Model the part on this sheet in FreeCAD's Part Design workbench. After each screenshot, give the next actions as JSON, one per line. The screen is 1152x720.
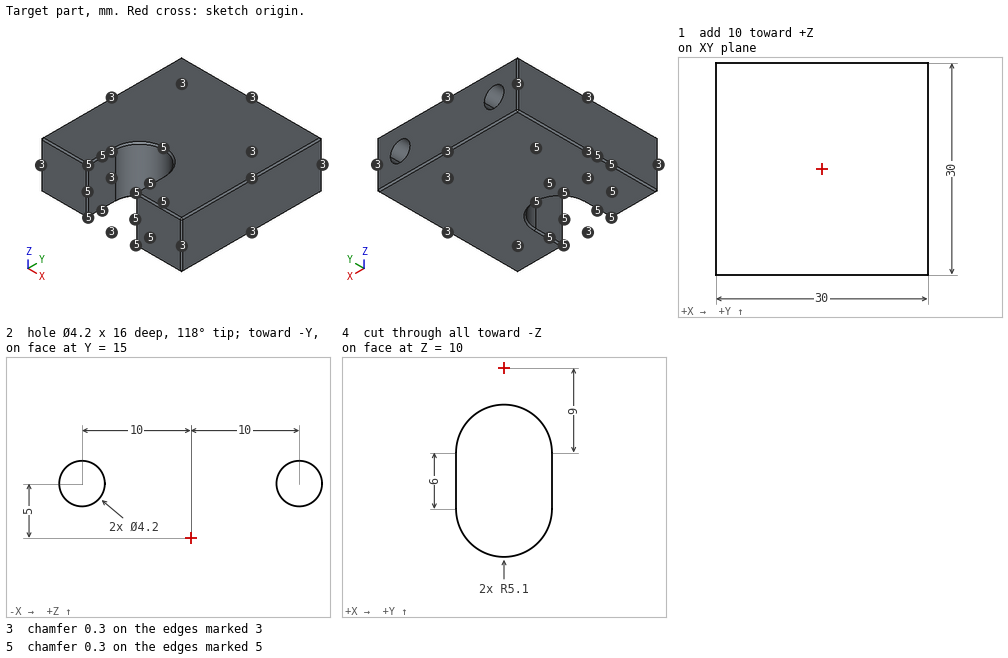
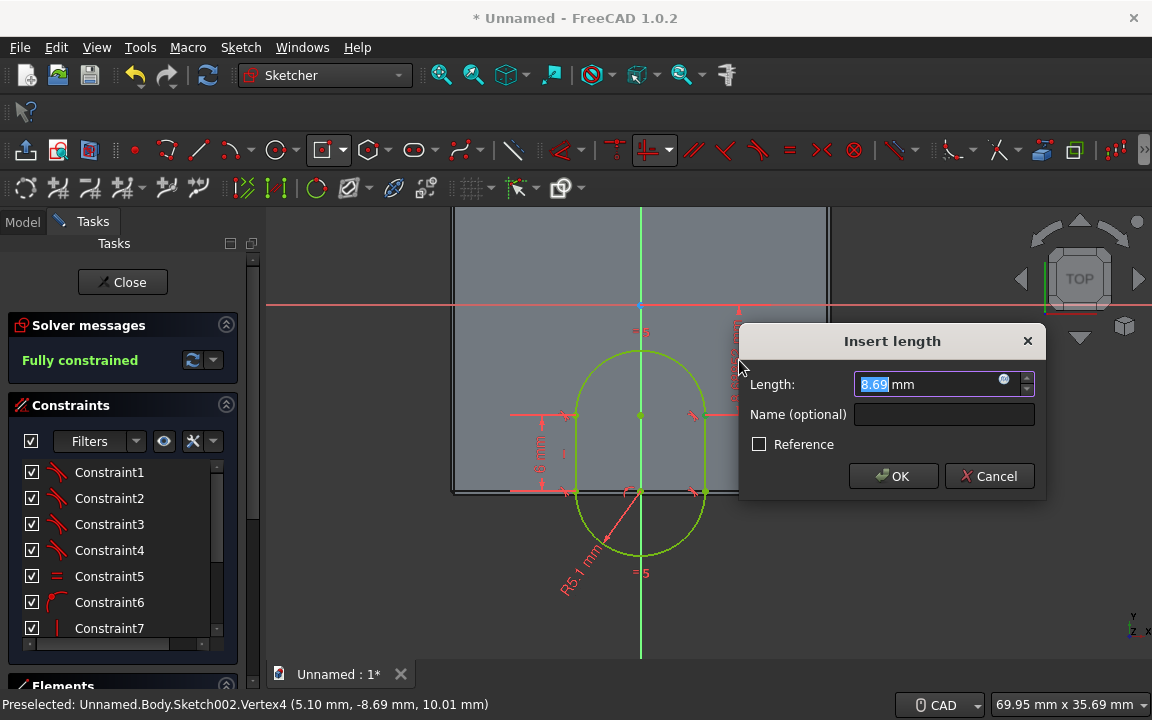
{"action": "type", "text": "9"}
{"action": "key", "text": "Return"}
{"action": "key", "text": "Escape"}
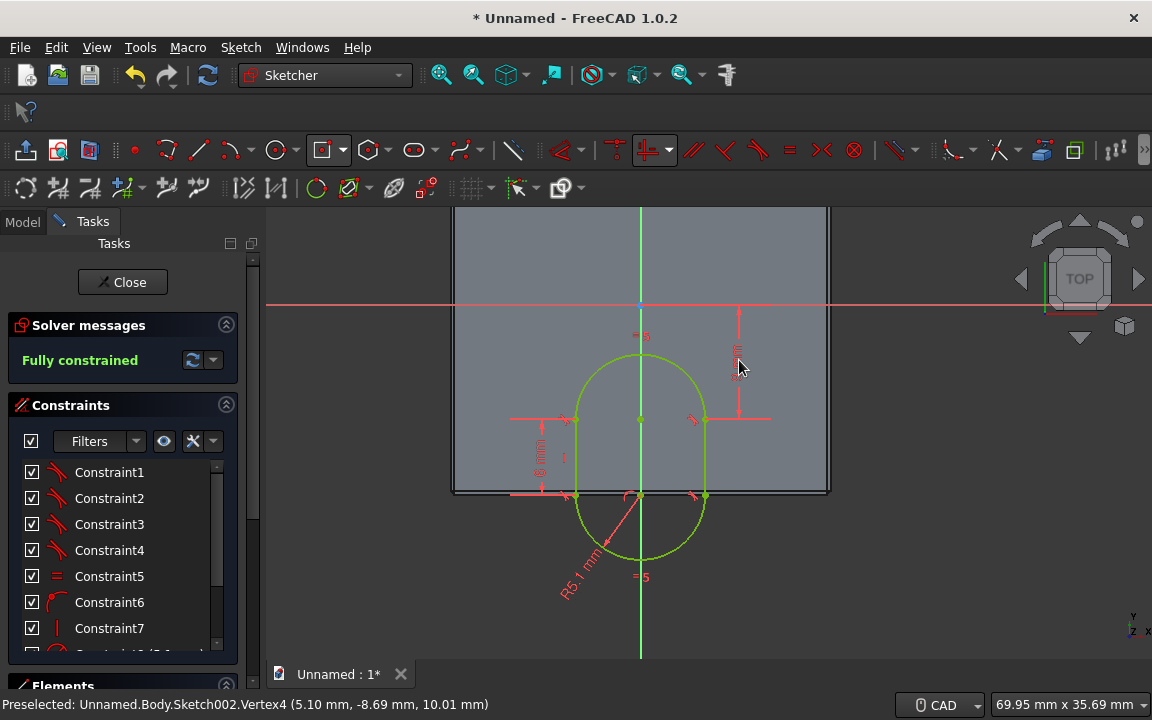
{"action": "left_click", "coordinate": [123, 282]}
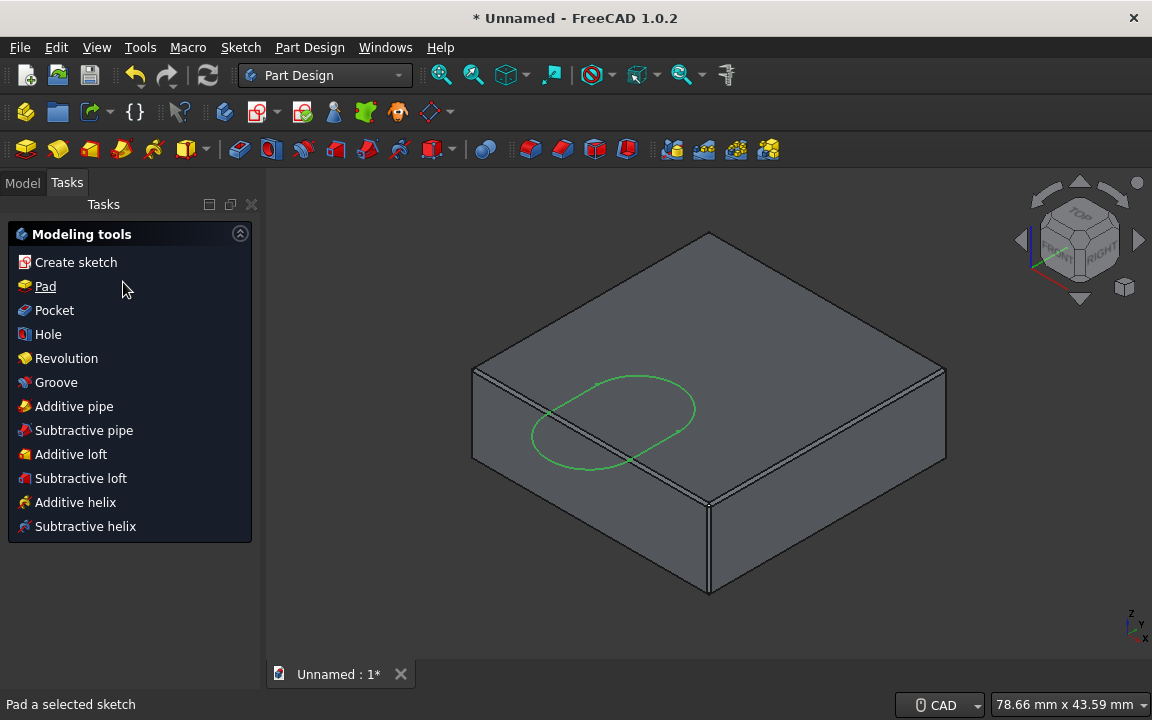
{"action": "left_click", "coordinate": [240, 150]}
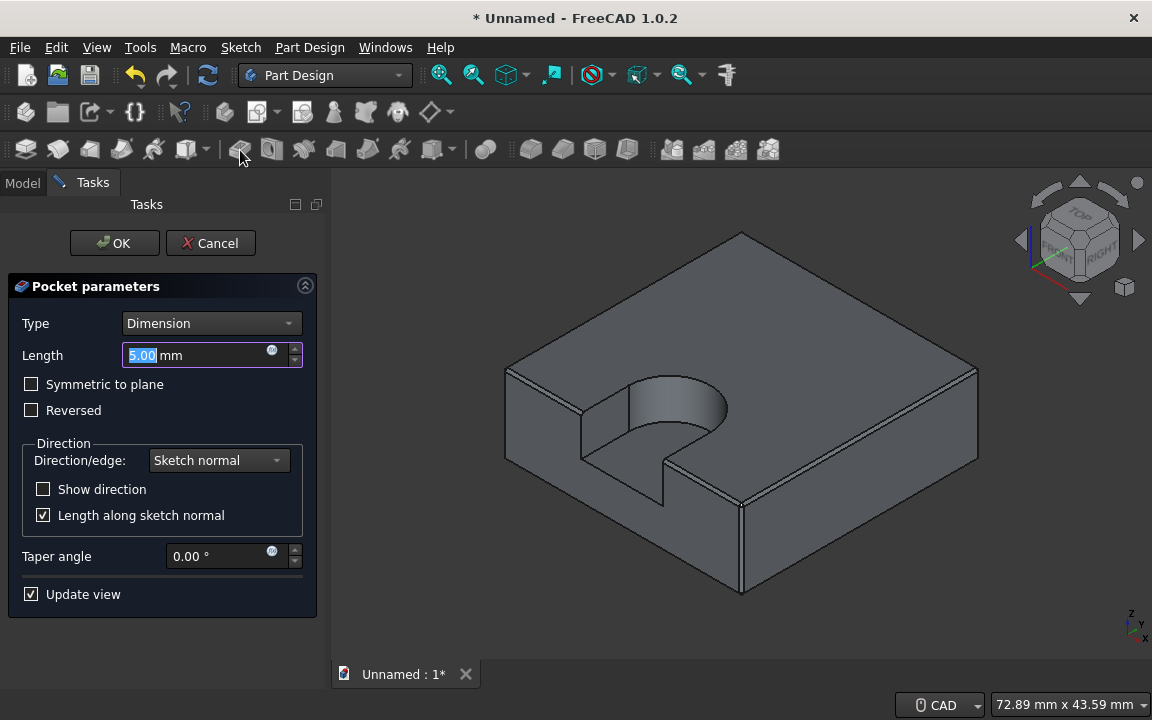
{"action": "left_click", "coordinate": [212, 324]}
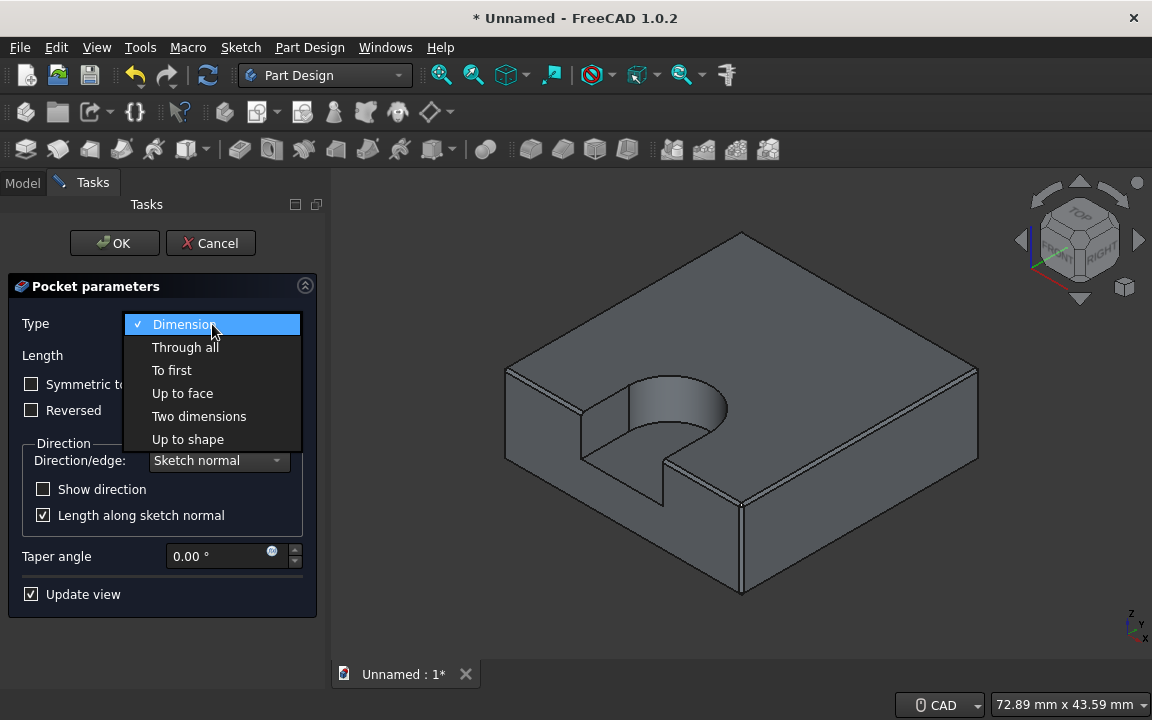
{"action": "left_click", "coordinate": [212, 348]}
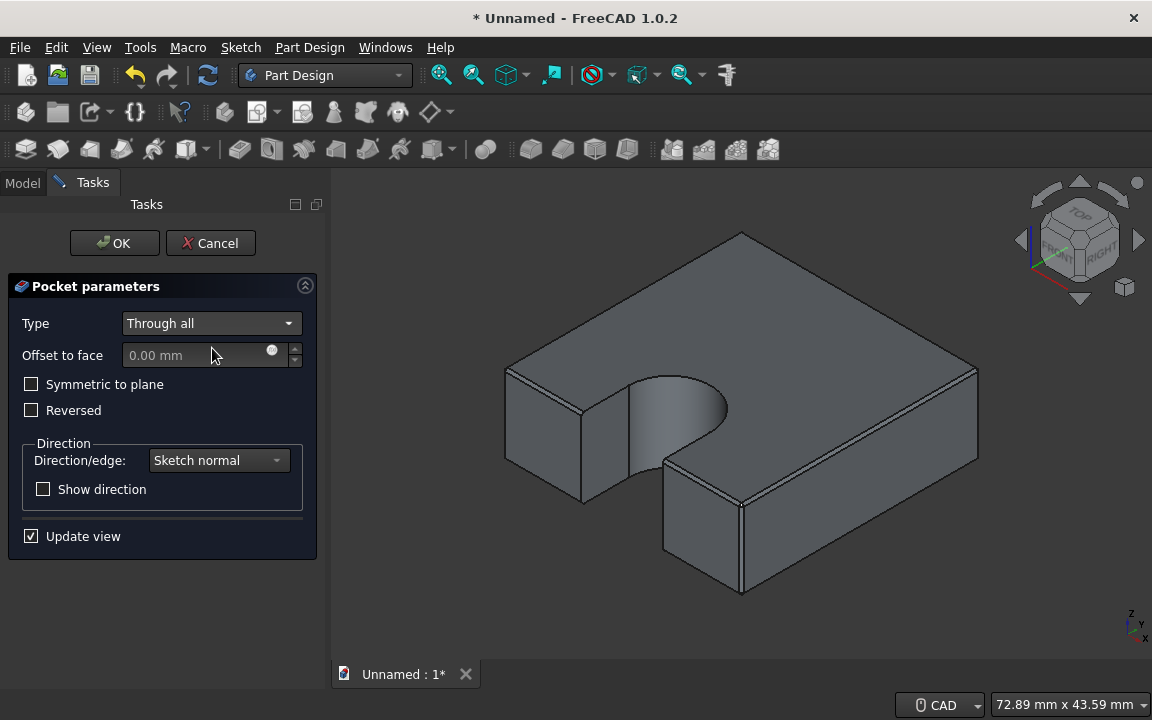
{"action": "left_click", "coordinate": [115, 243]}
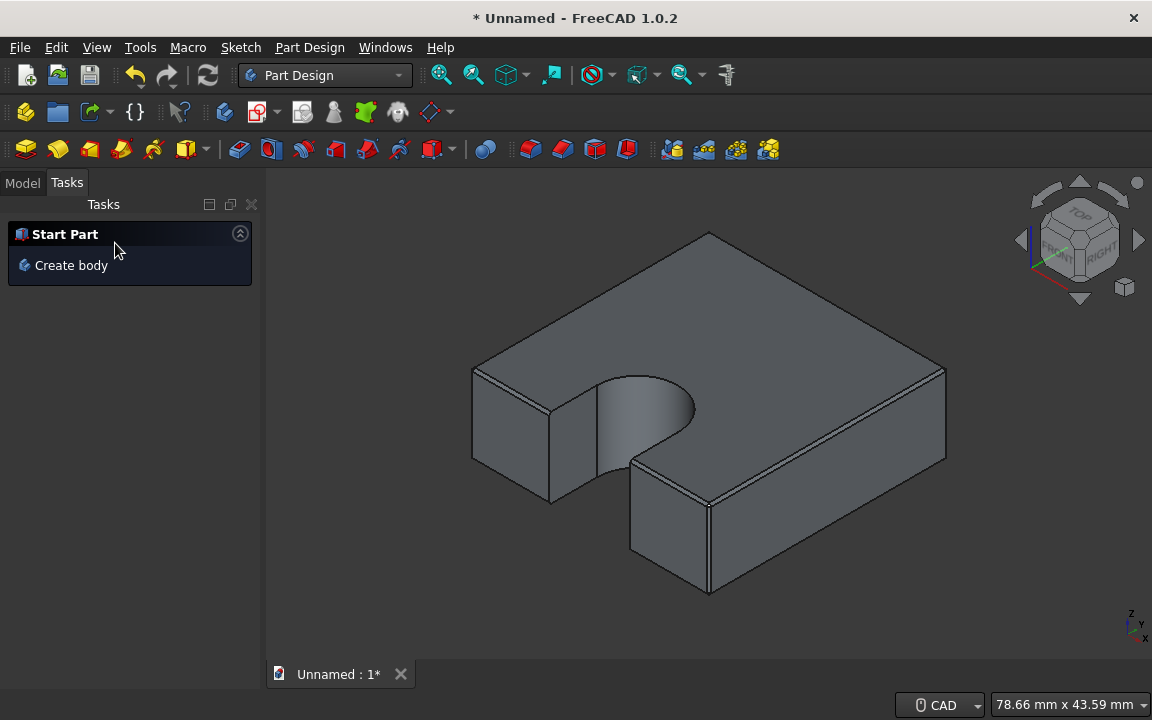
{"action": "left_click", "coordinate": [549, 458]}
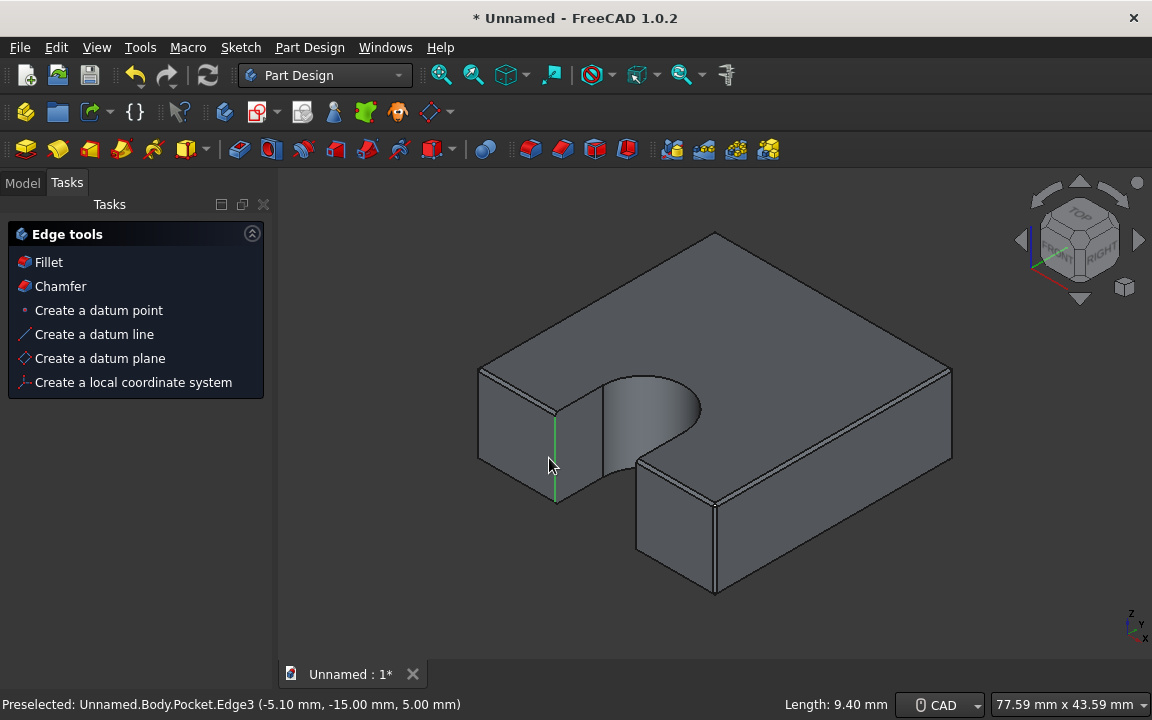
{"action": "left_click", "coordinate": [684, 384], "text": "ctrl"}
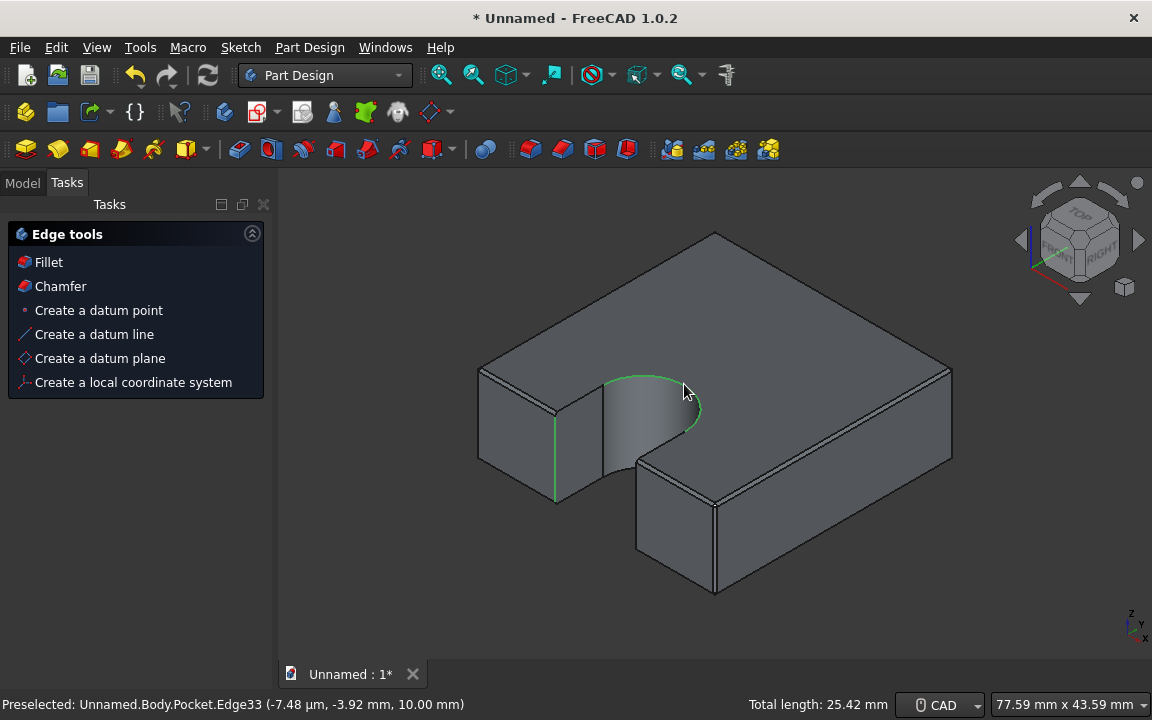
{"action": "left_click", "coordinate": [580, 398], "text": "ctrl"}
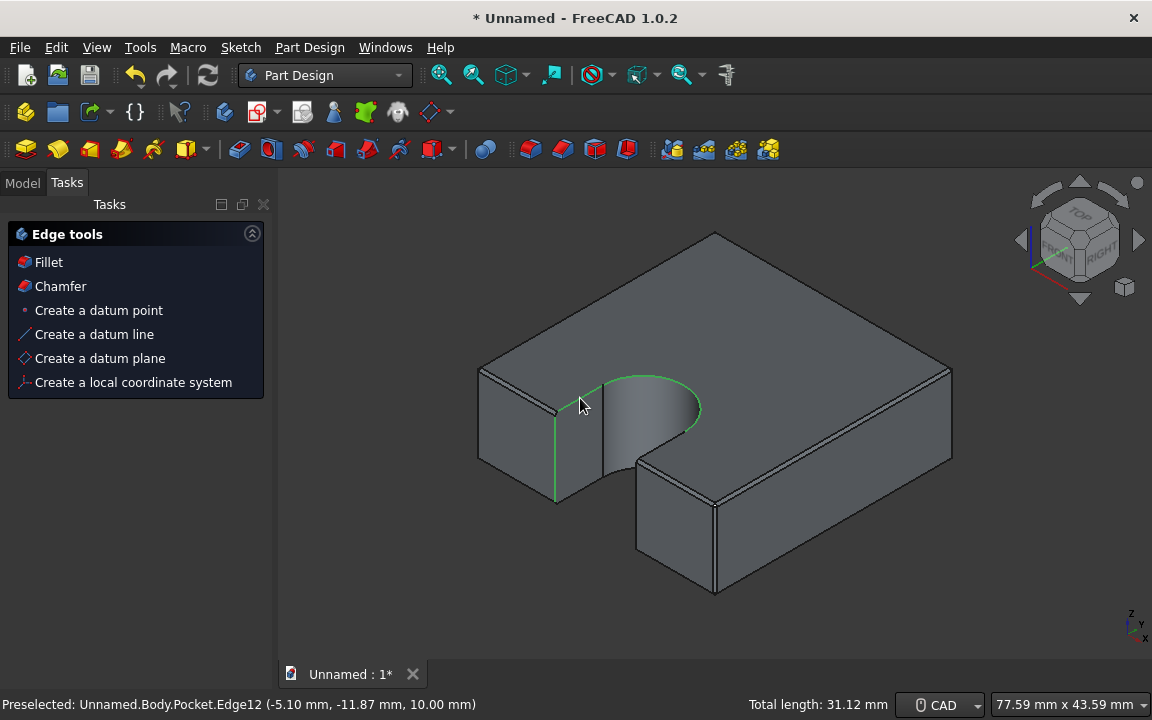
{"action": "scroll", "coordinate": [637, 549], "scroll_direction": "up", "scroll_amount": 11}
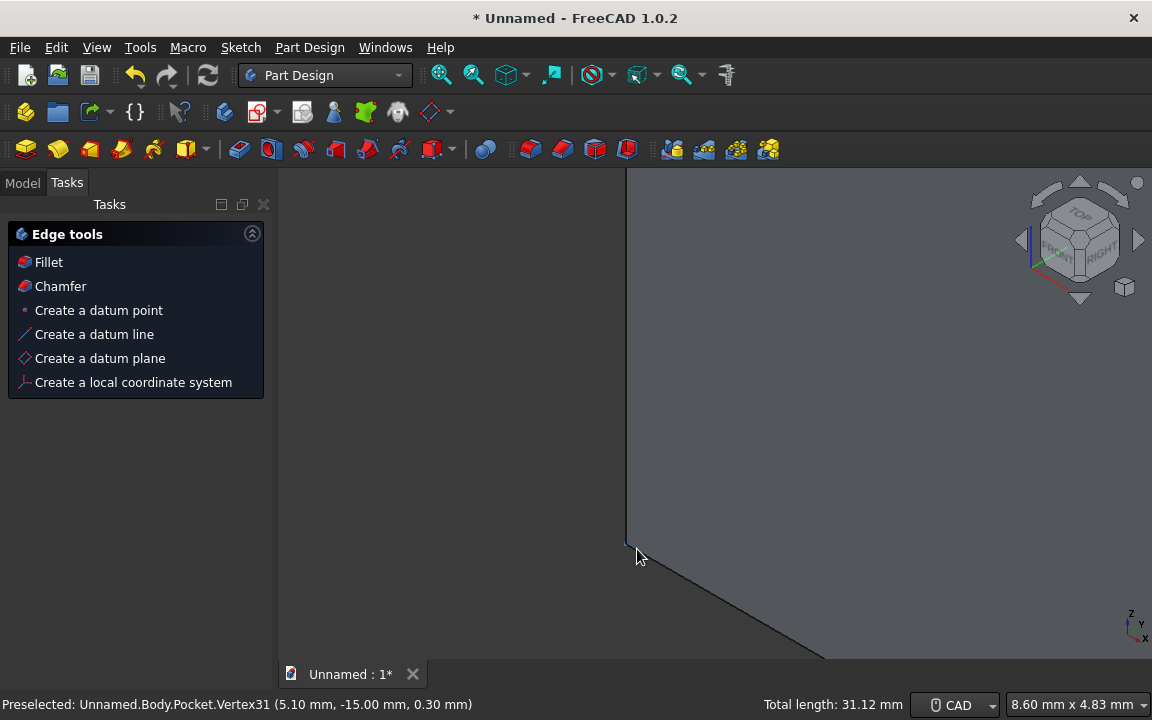
{"action": "left_click", "coordinate": [442, 76]}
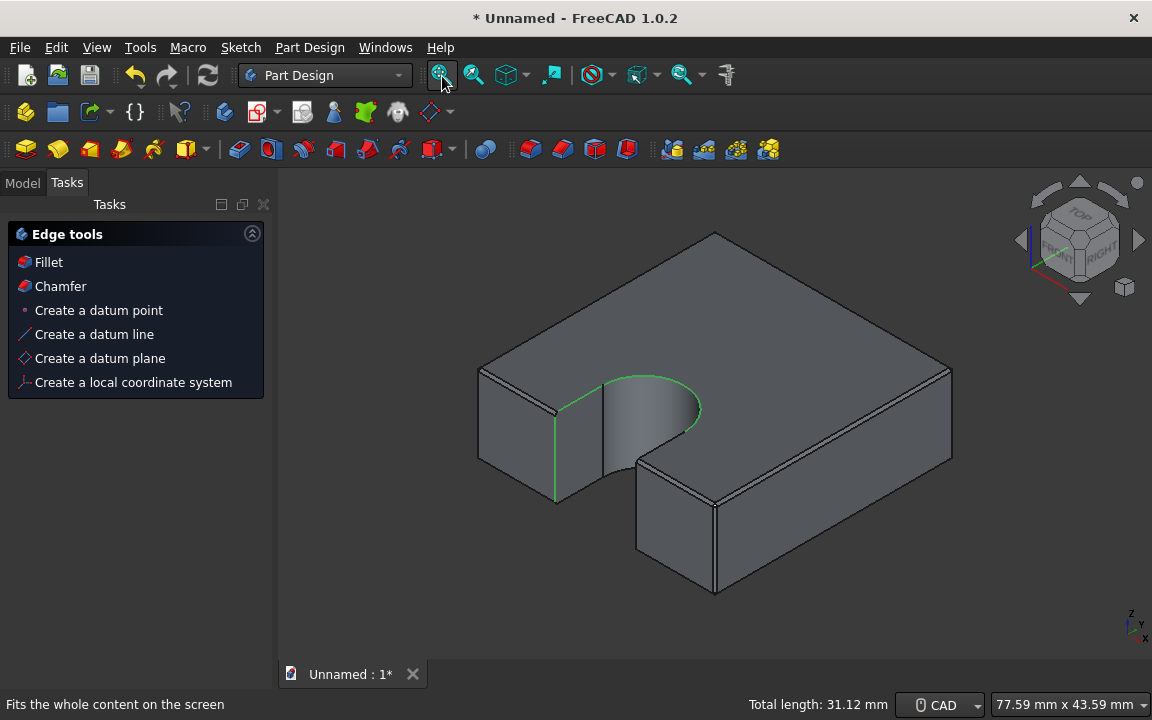
{"action": "key", "text": "2"}